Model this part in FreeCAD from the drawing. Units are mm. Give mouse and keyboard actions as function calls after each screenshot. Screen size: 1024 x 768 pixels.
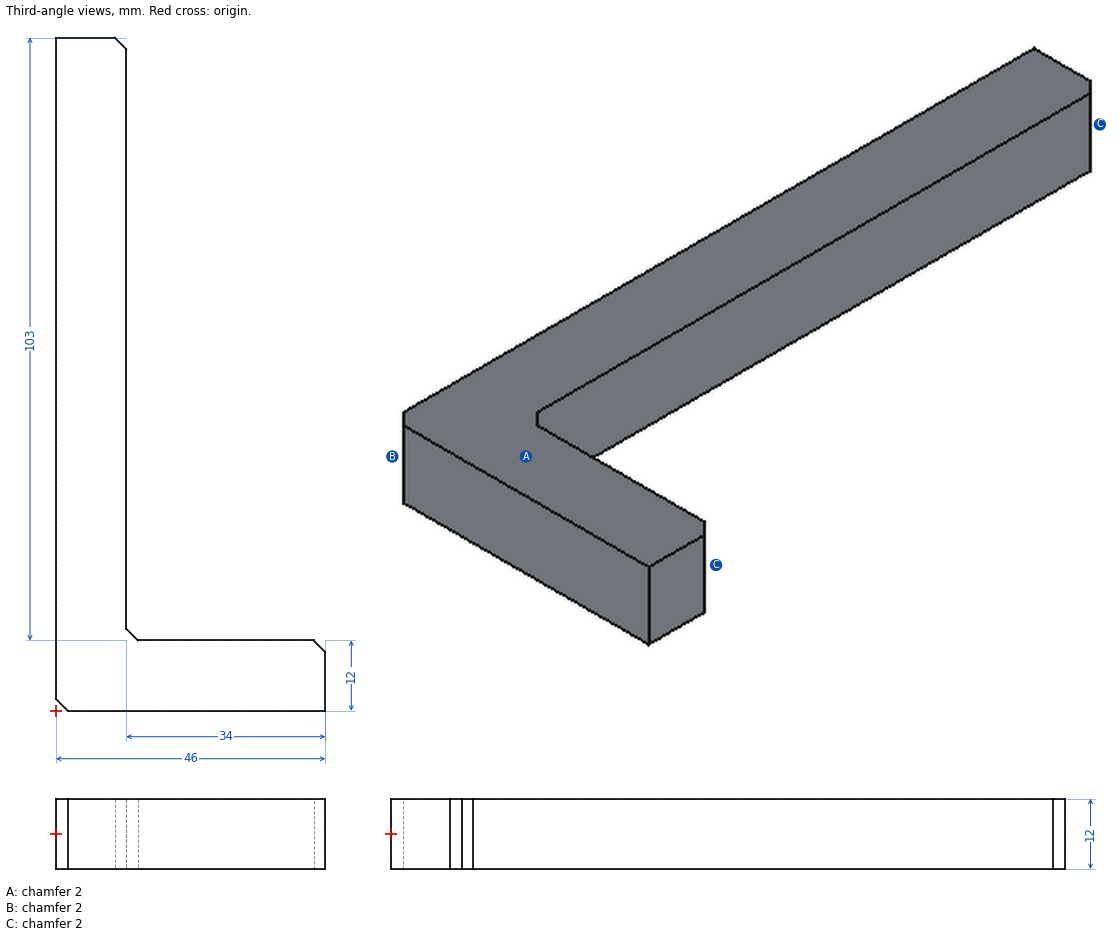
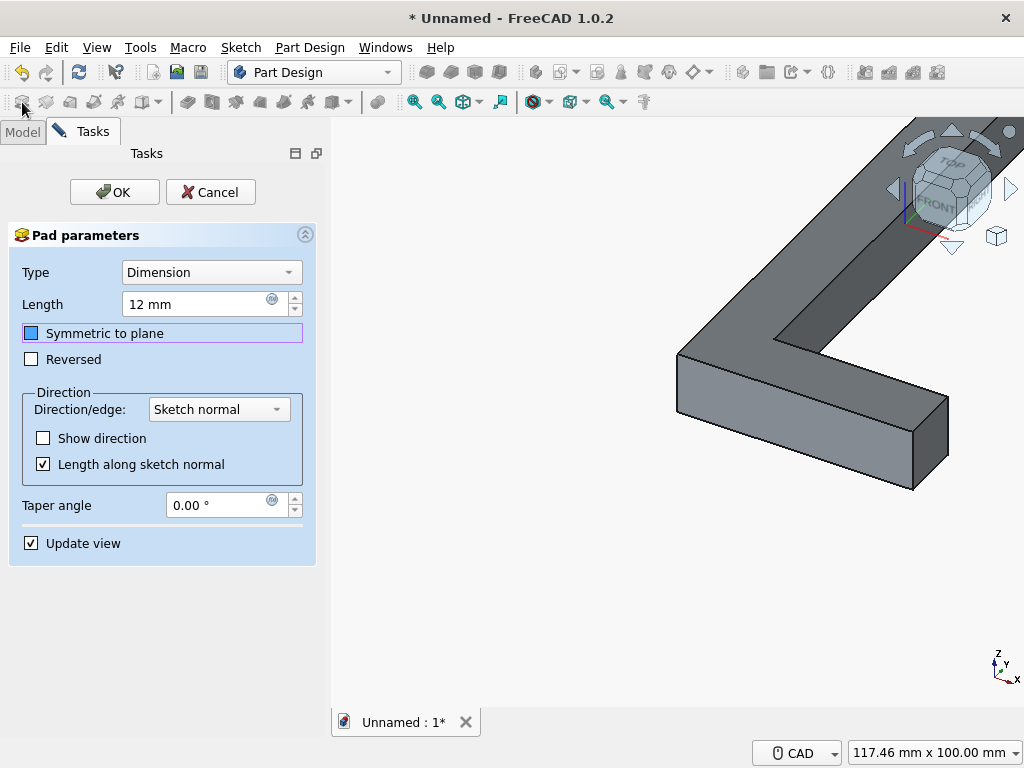
click(30, 333)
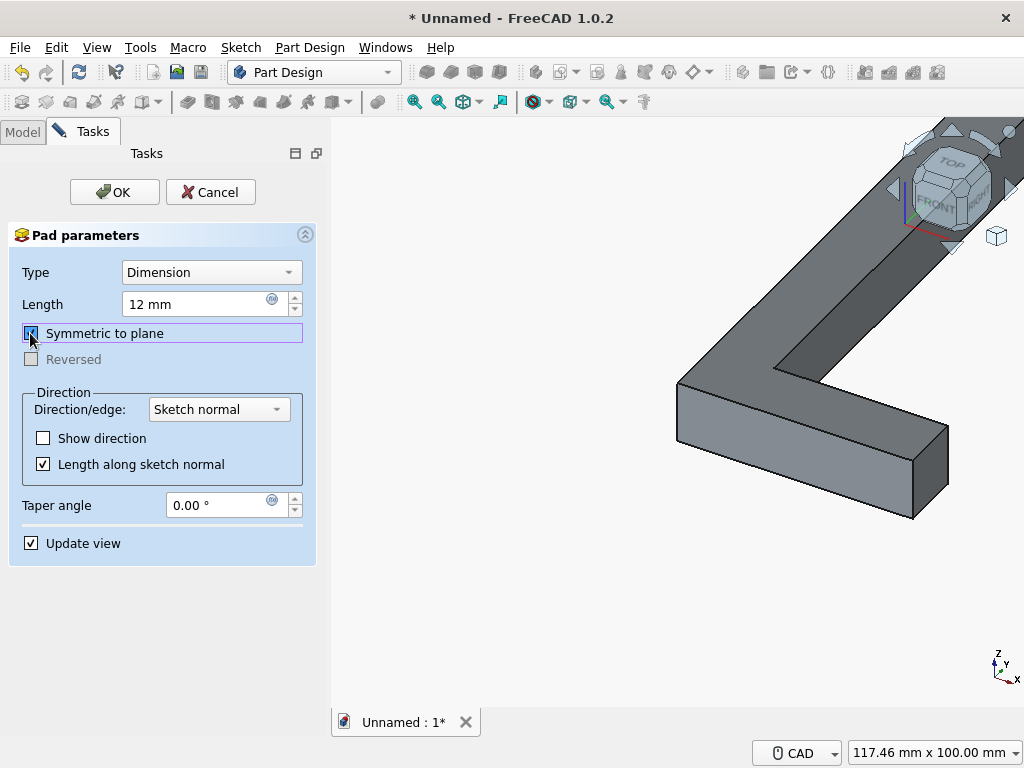
click(115, 192)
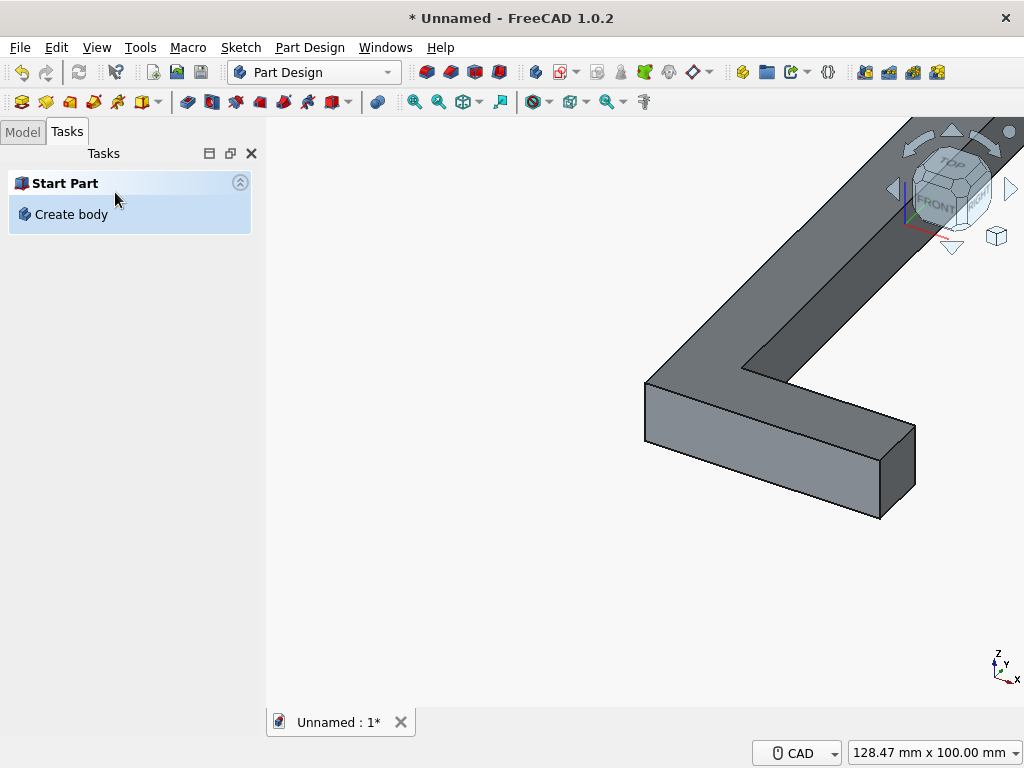
click(416, 102)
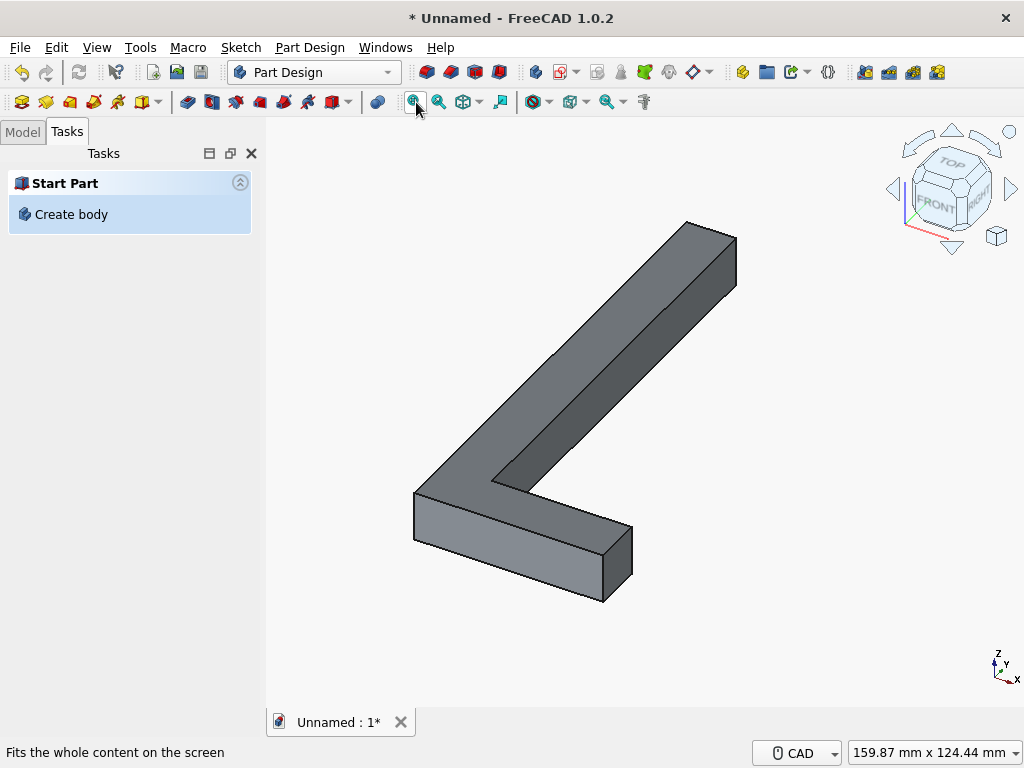
key(0)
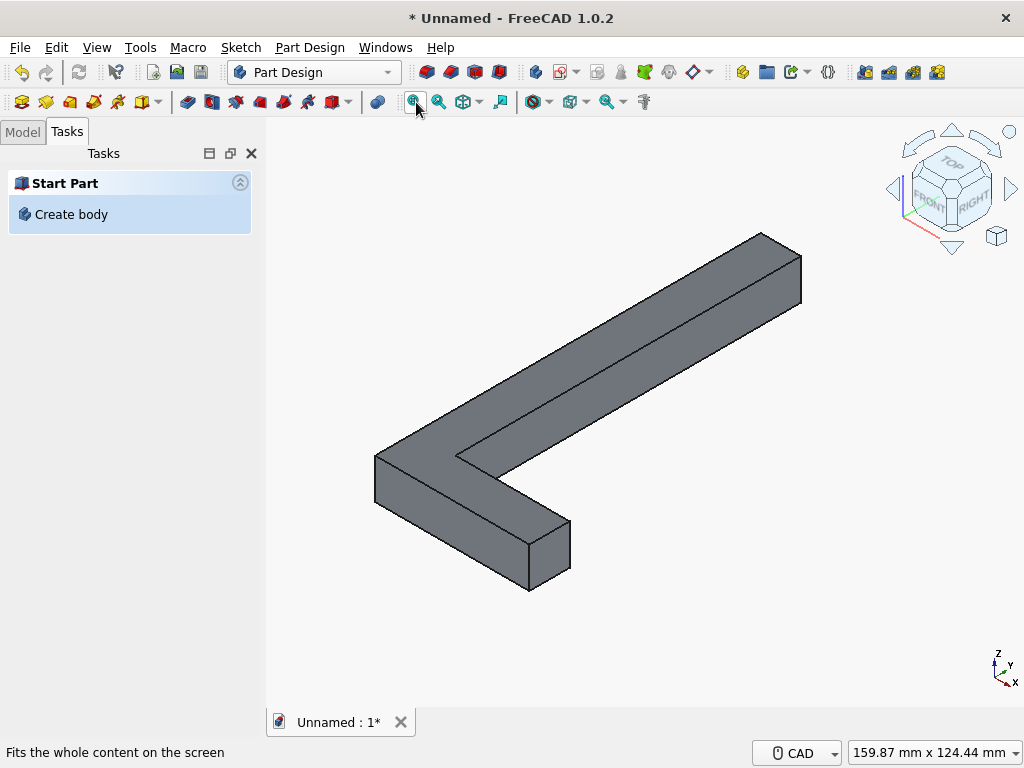
key(2)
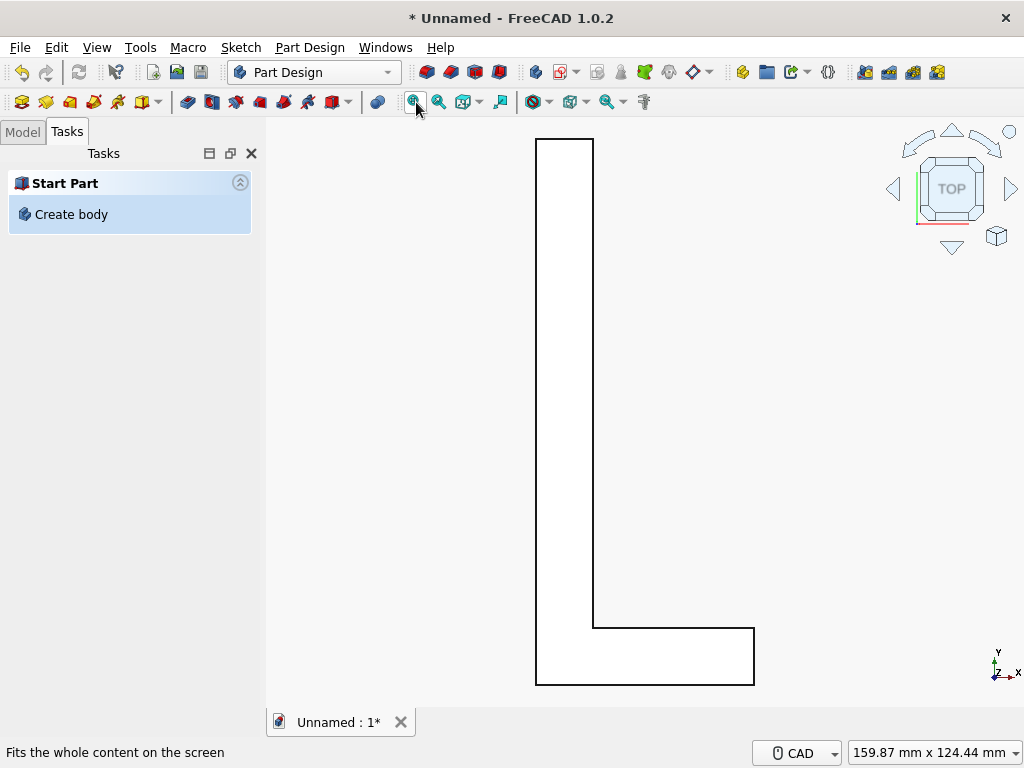
key(1)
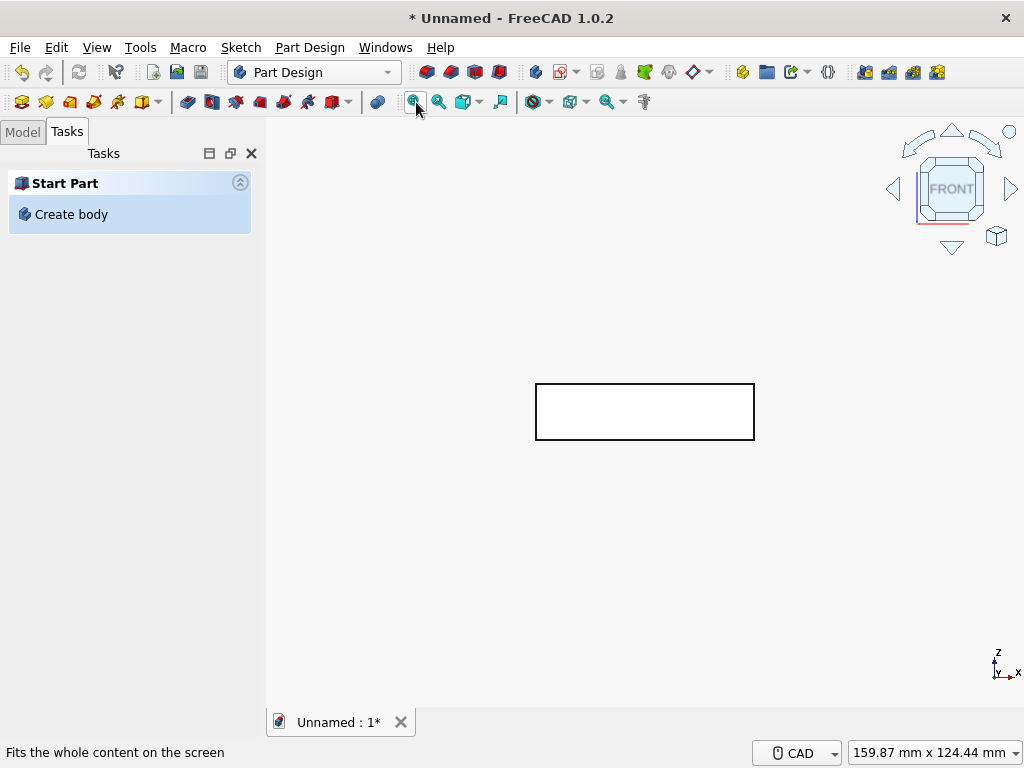
click(416, 102)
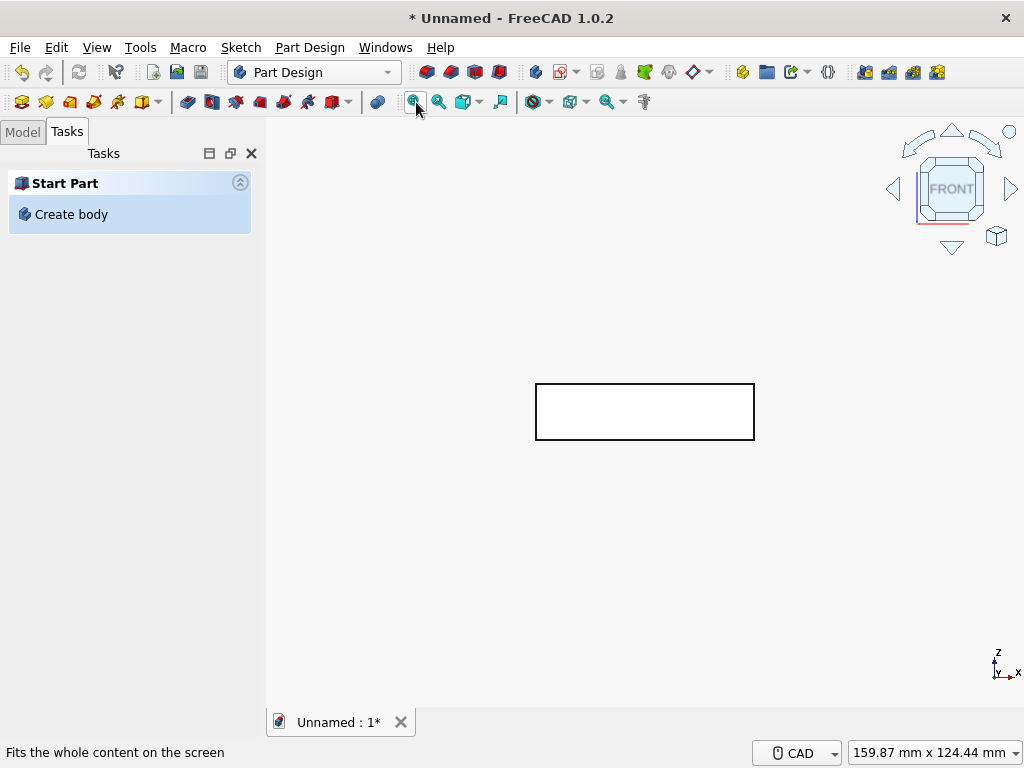
key(3)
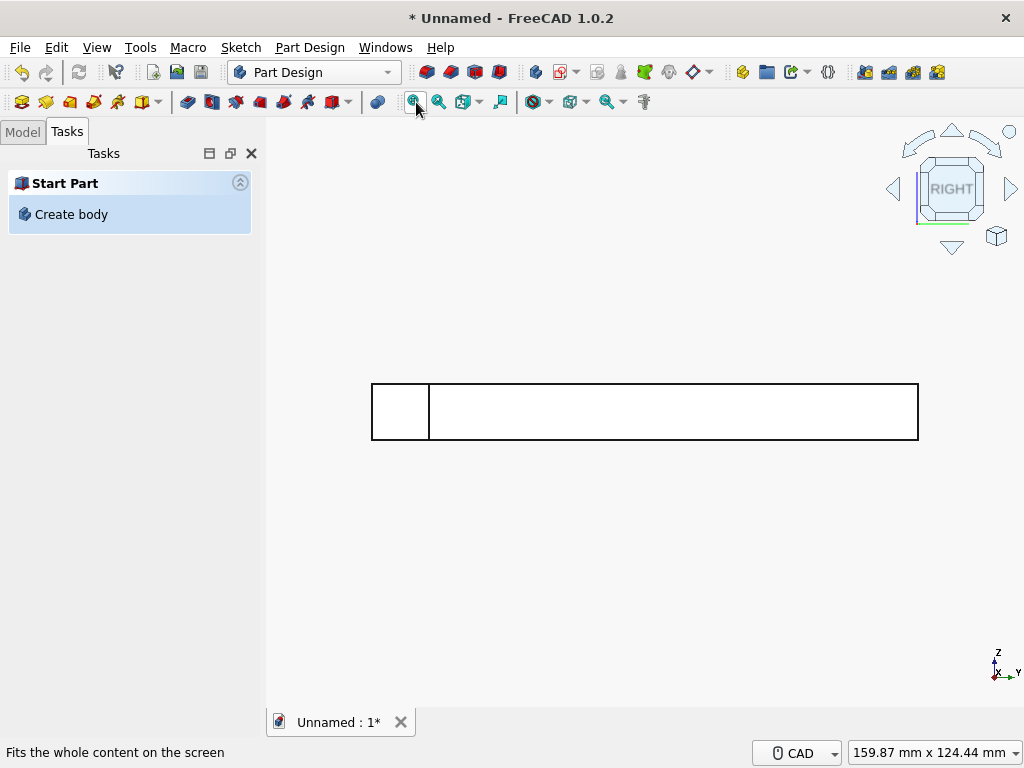
key(5)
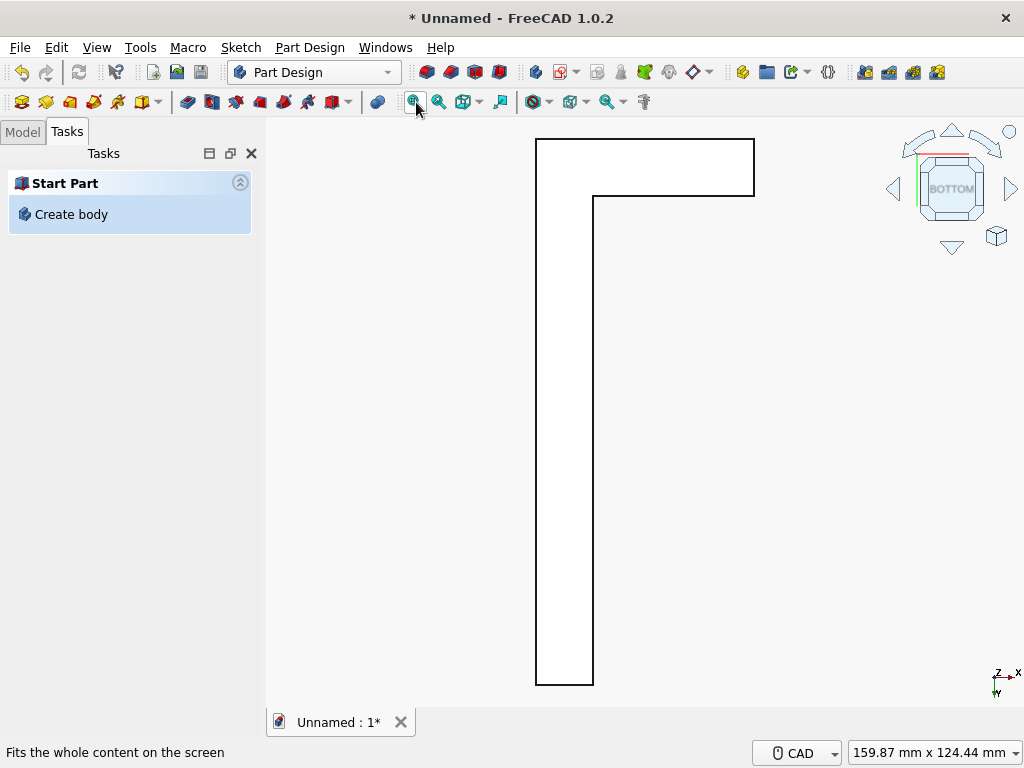
key(4)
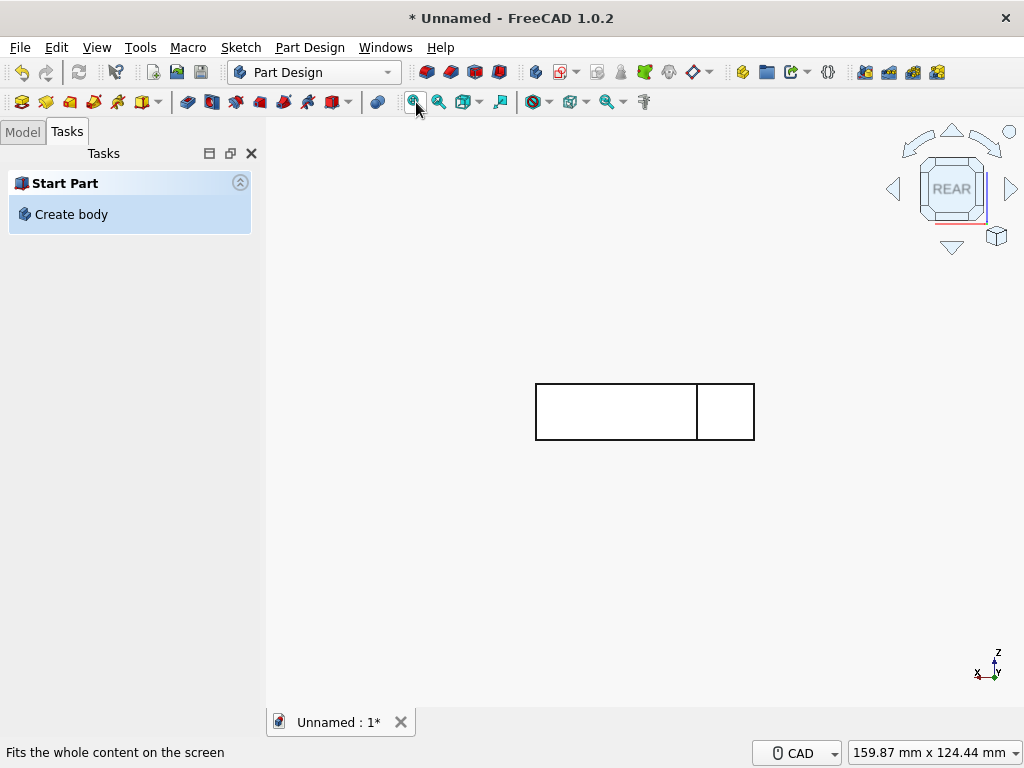
click(416, 102)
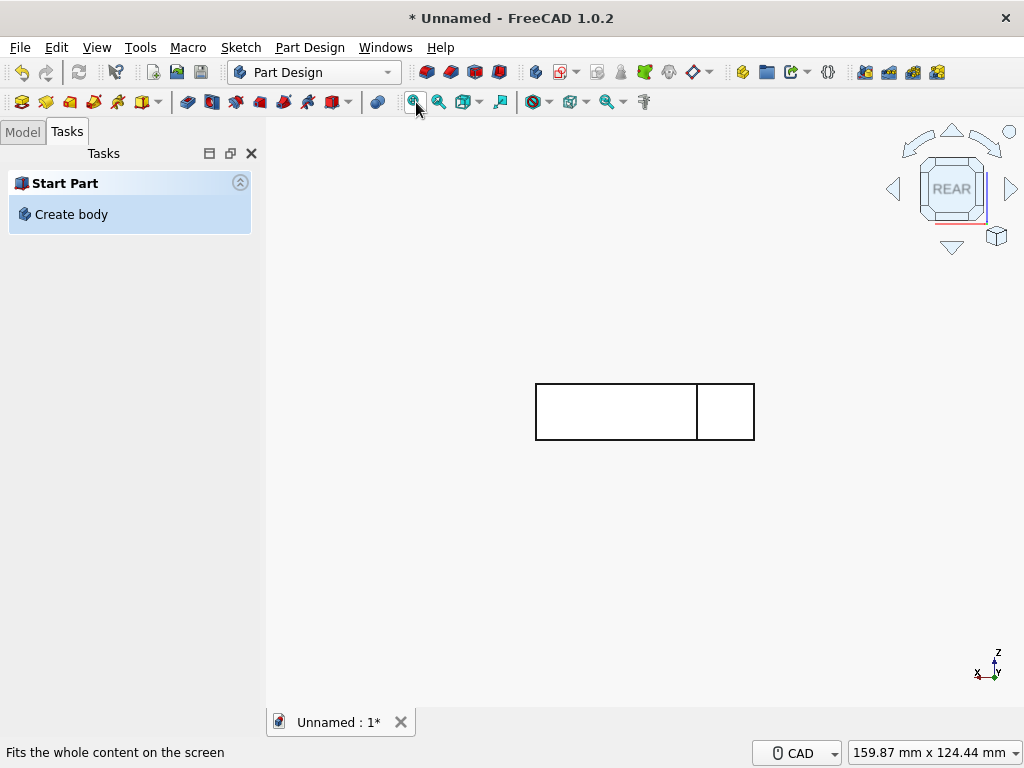
key(6)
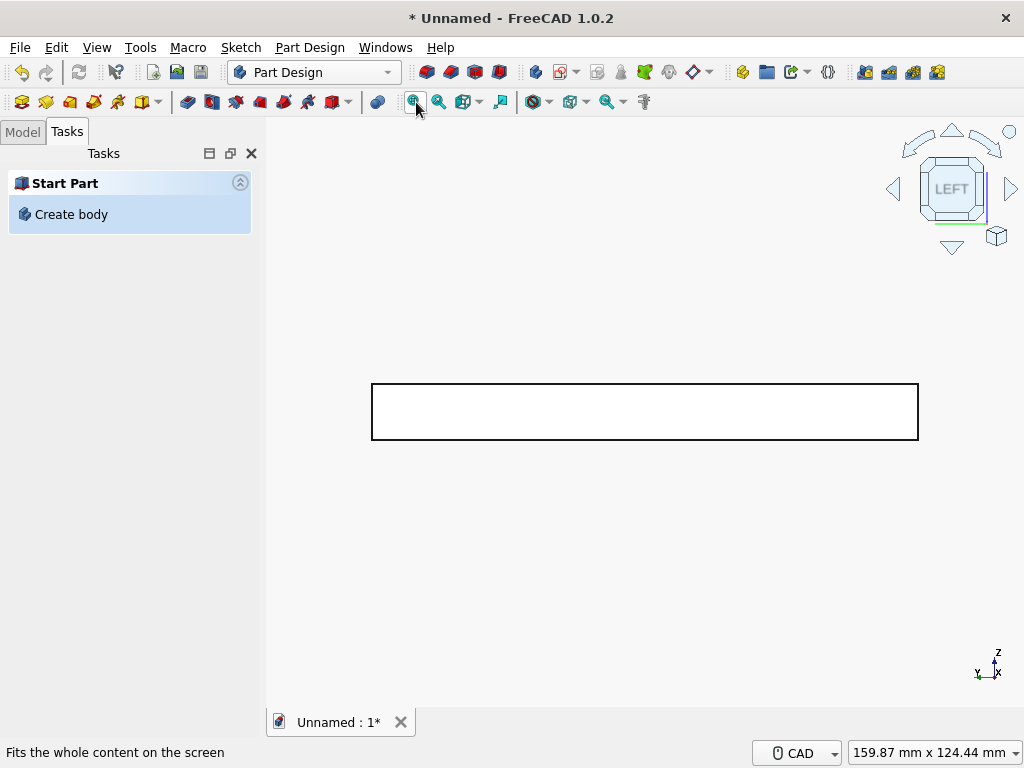
key(v)
key(3)